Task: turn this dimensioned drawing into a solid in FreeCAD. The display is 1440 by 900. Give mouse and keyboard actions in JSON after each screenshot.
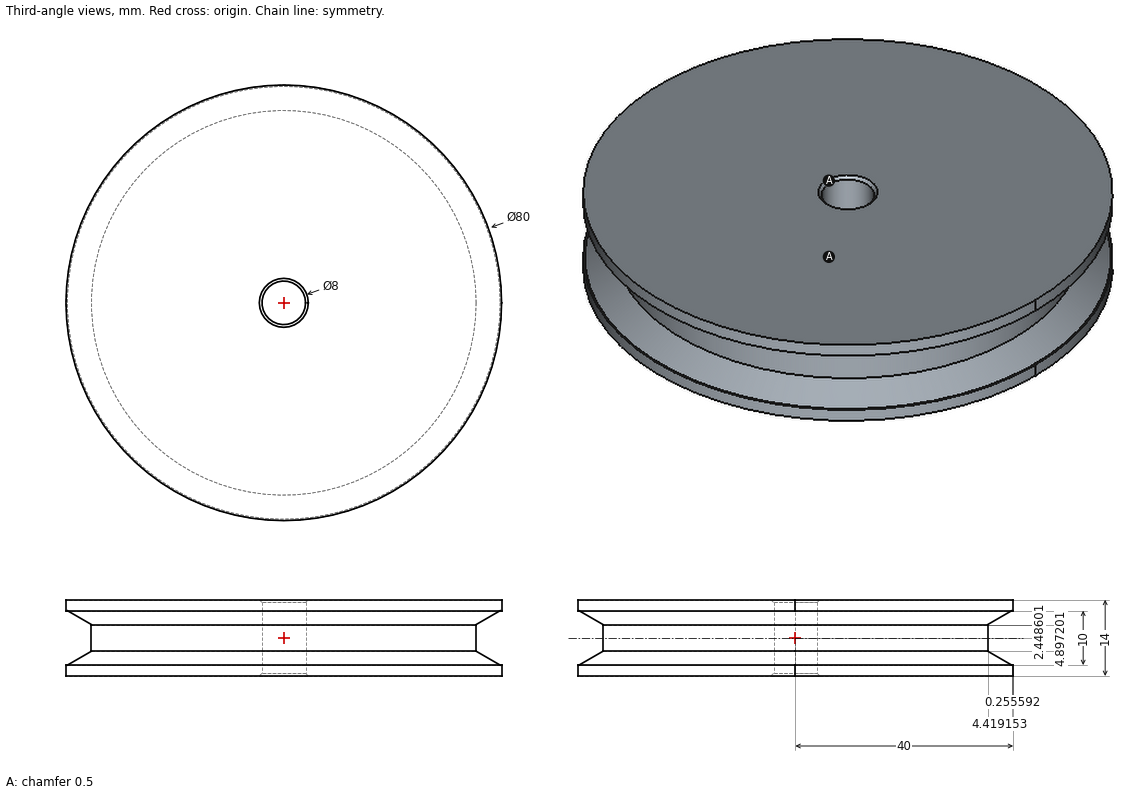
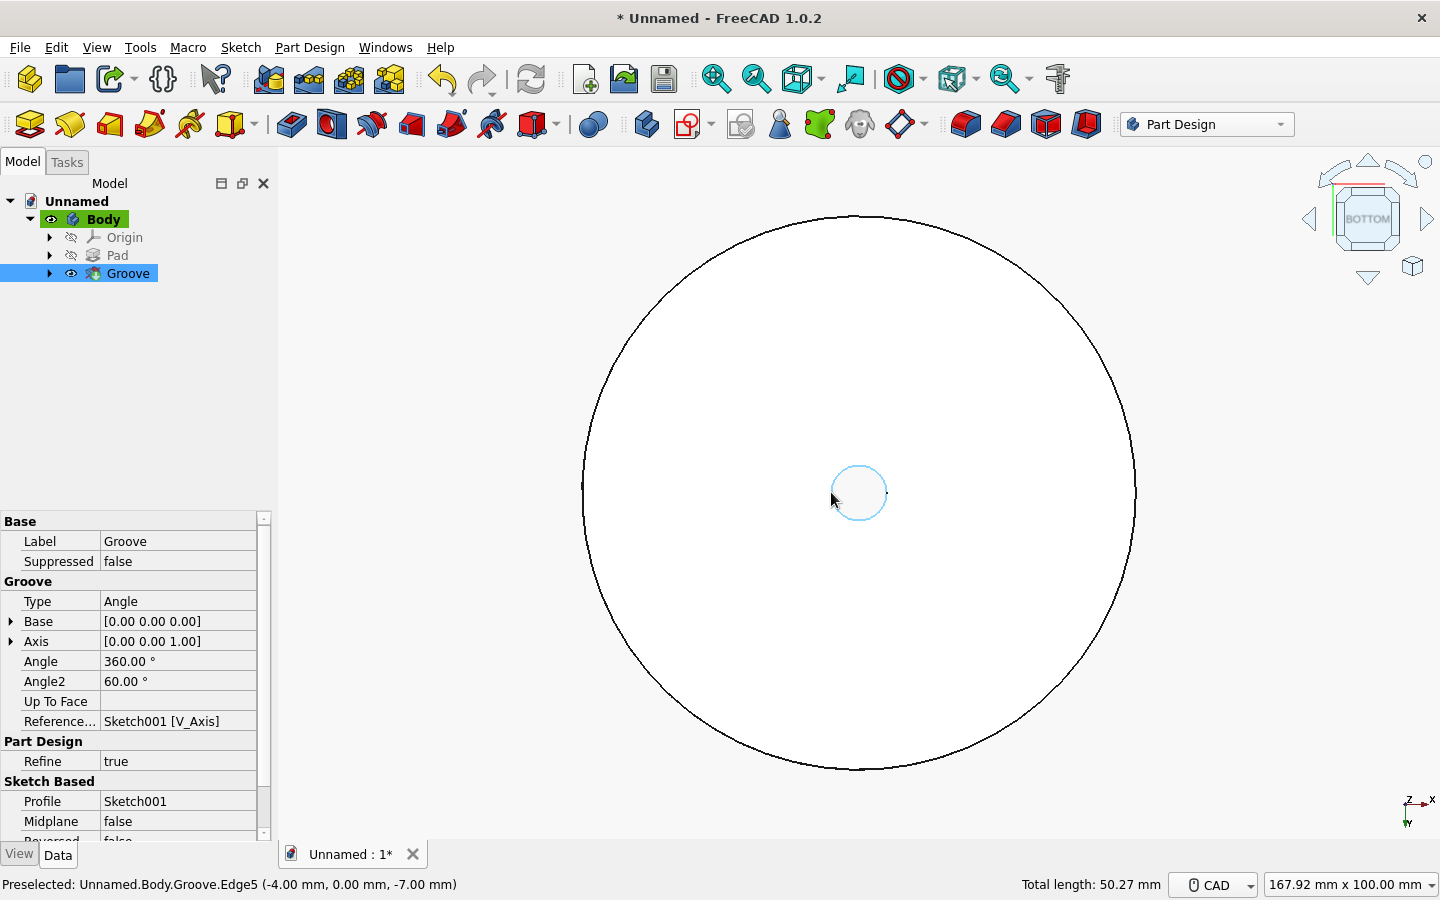
{"action": "left_click", "coordinate": [1006, 124]}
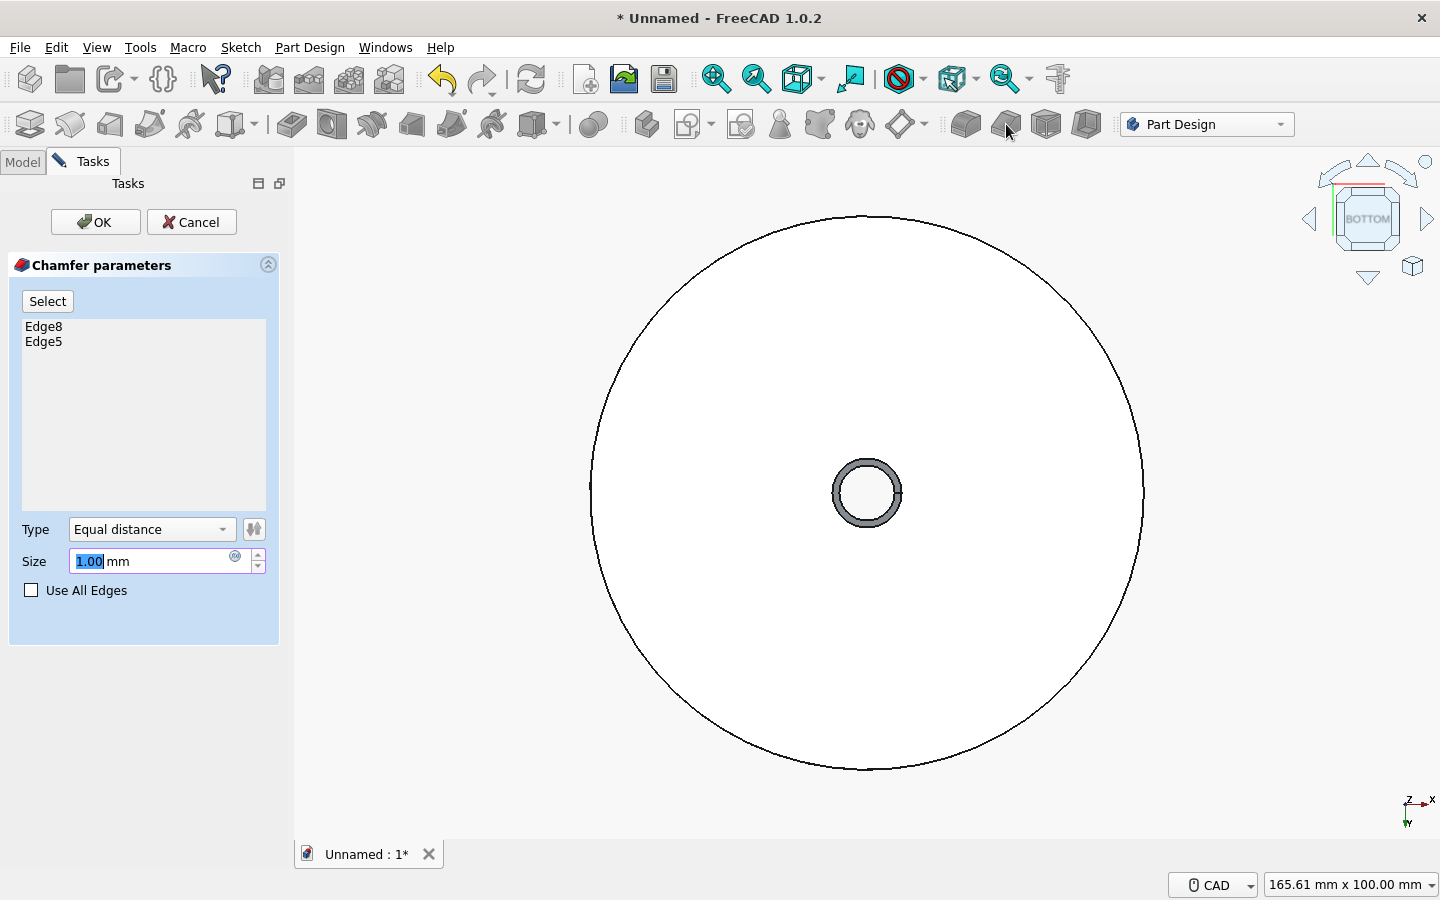
{"action": "type", "text": "0.5"}
{"action": "key", "text": "Tab"}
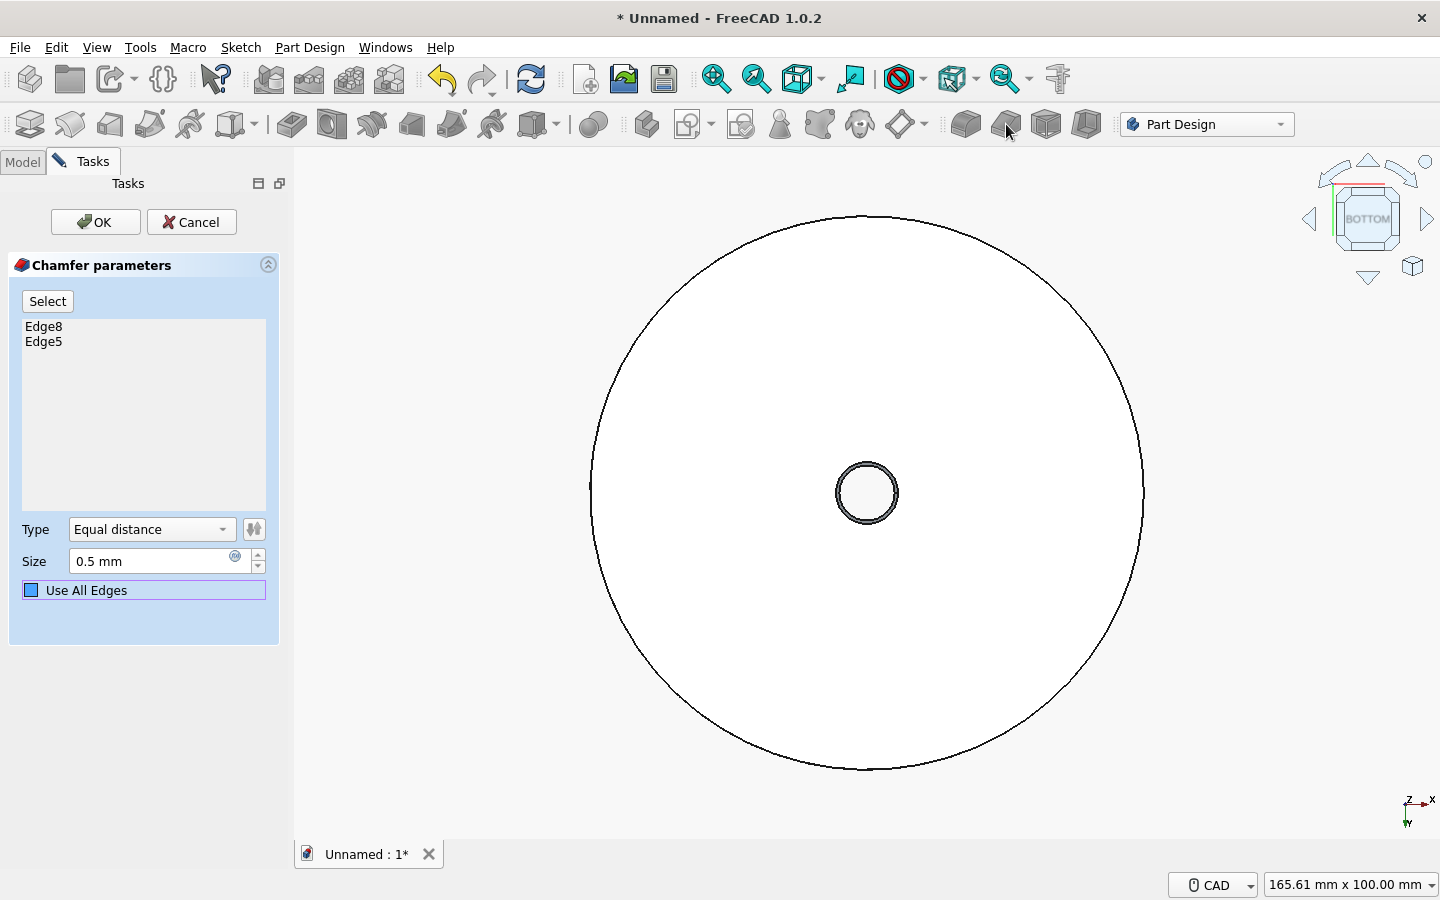
{"action": "left_click", "coordinate": [96, 222]}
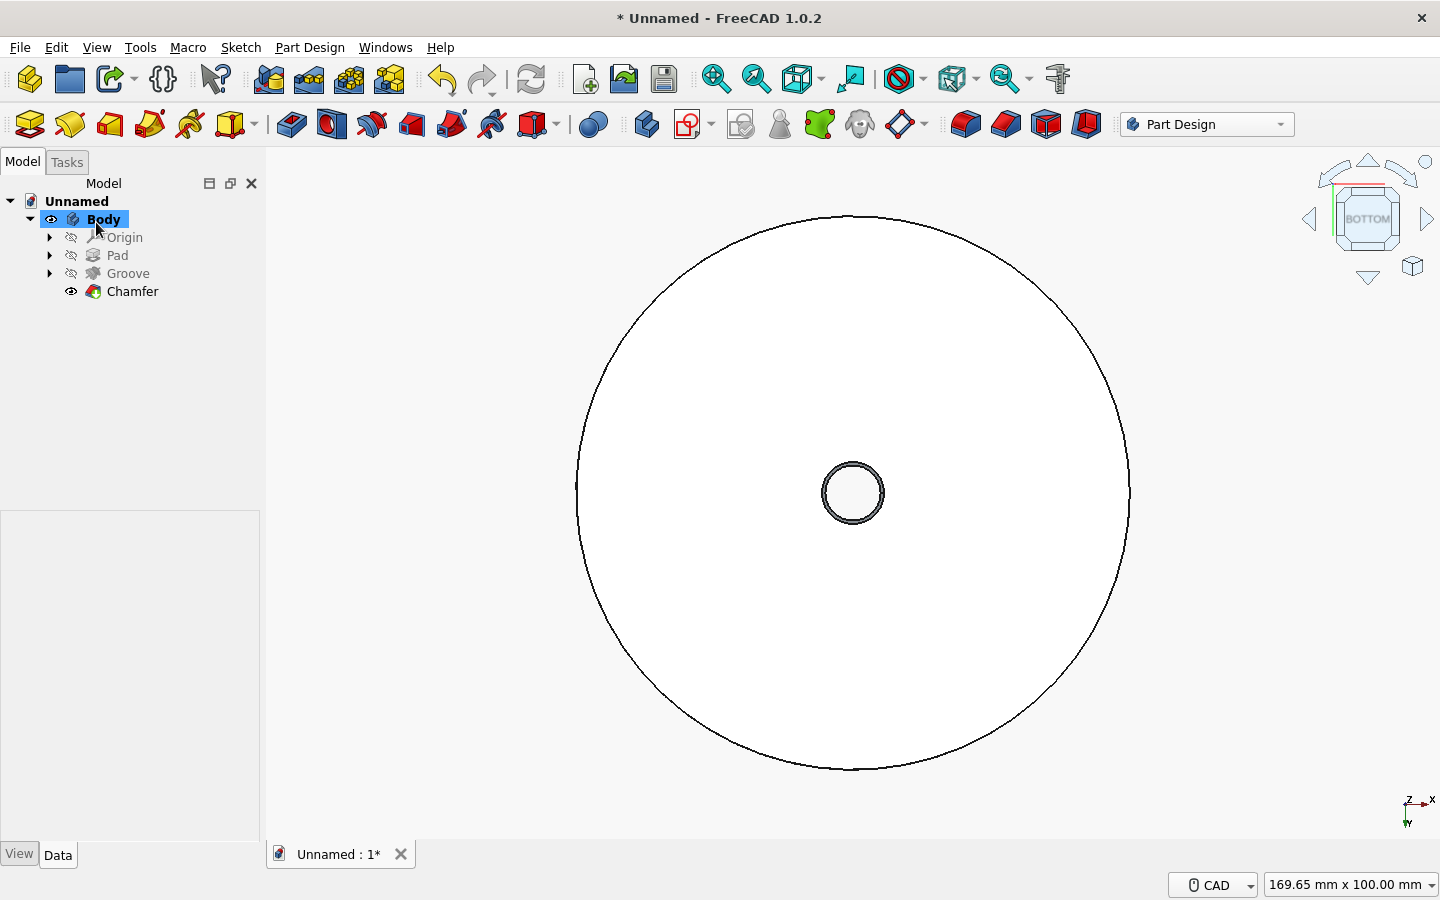
{"action": "key", "text": "0"}